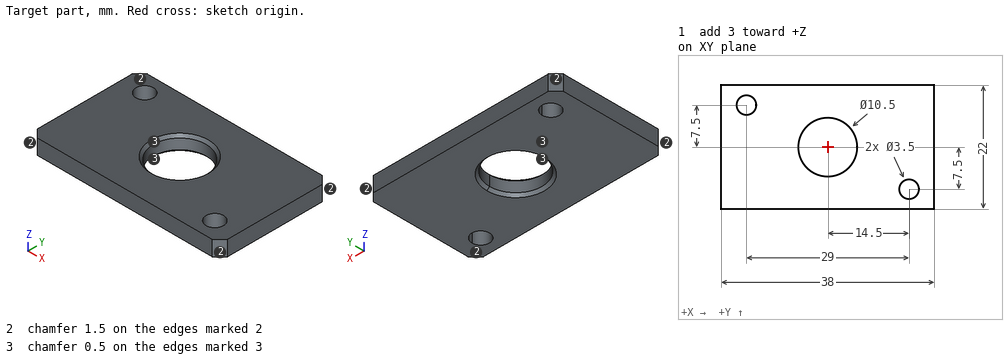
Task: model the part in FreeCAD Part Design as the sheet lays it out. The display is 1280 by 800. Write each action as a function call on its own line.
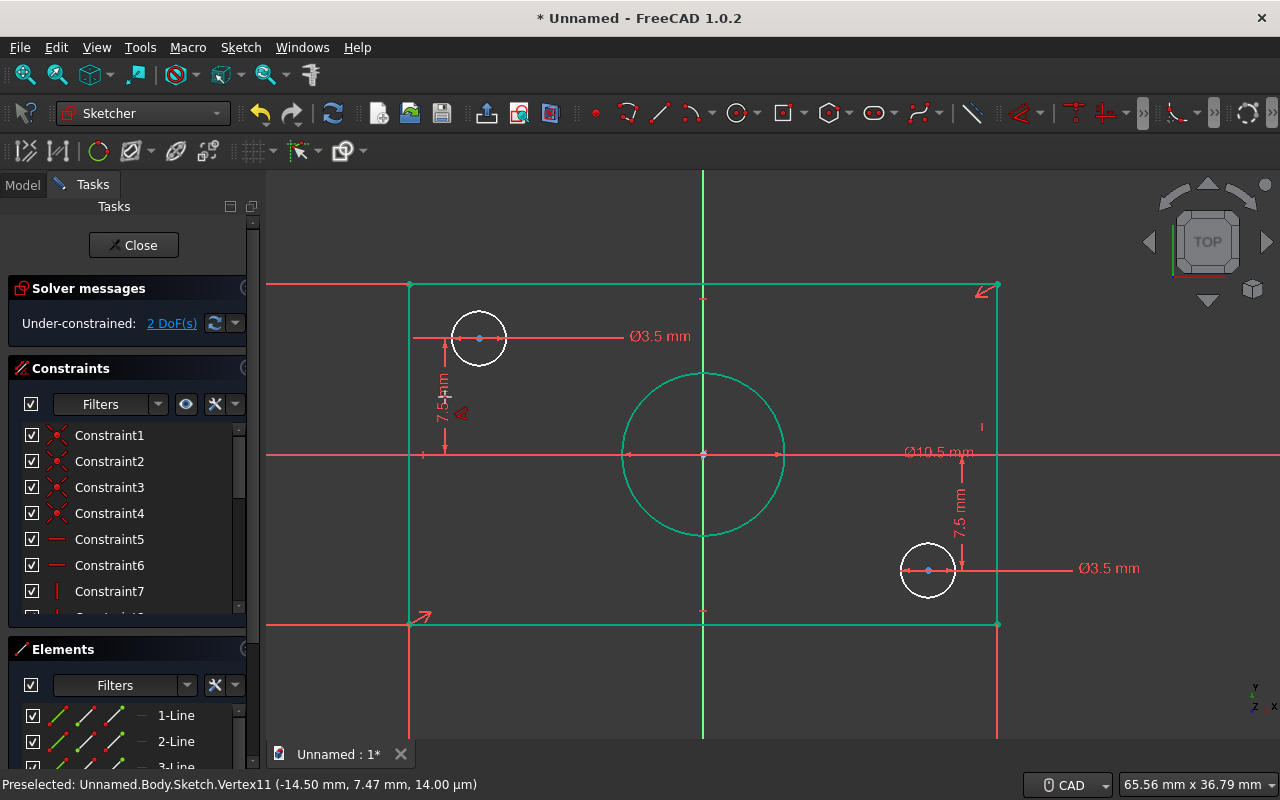
click(928, 571)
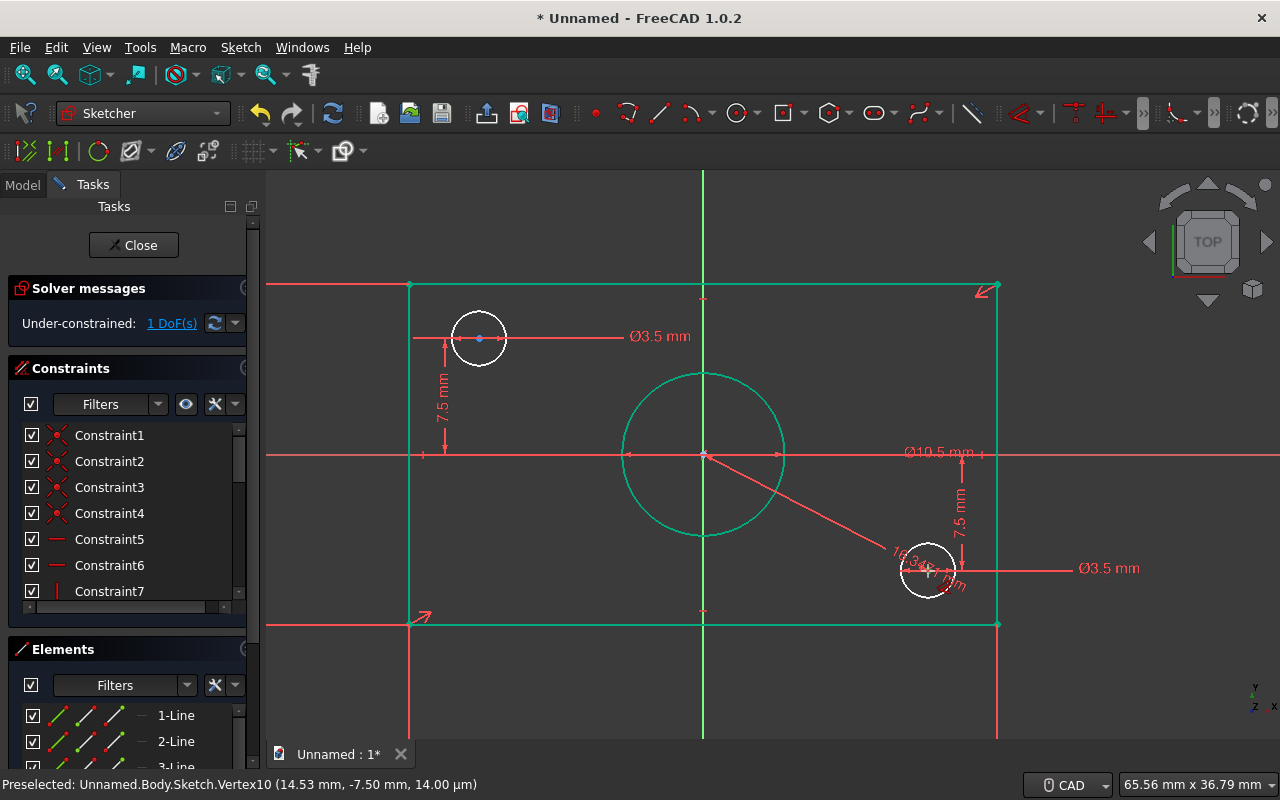
click(479, 338)
click(600, 605)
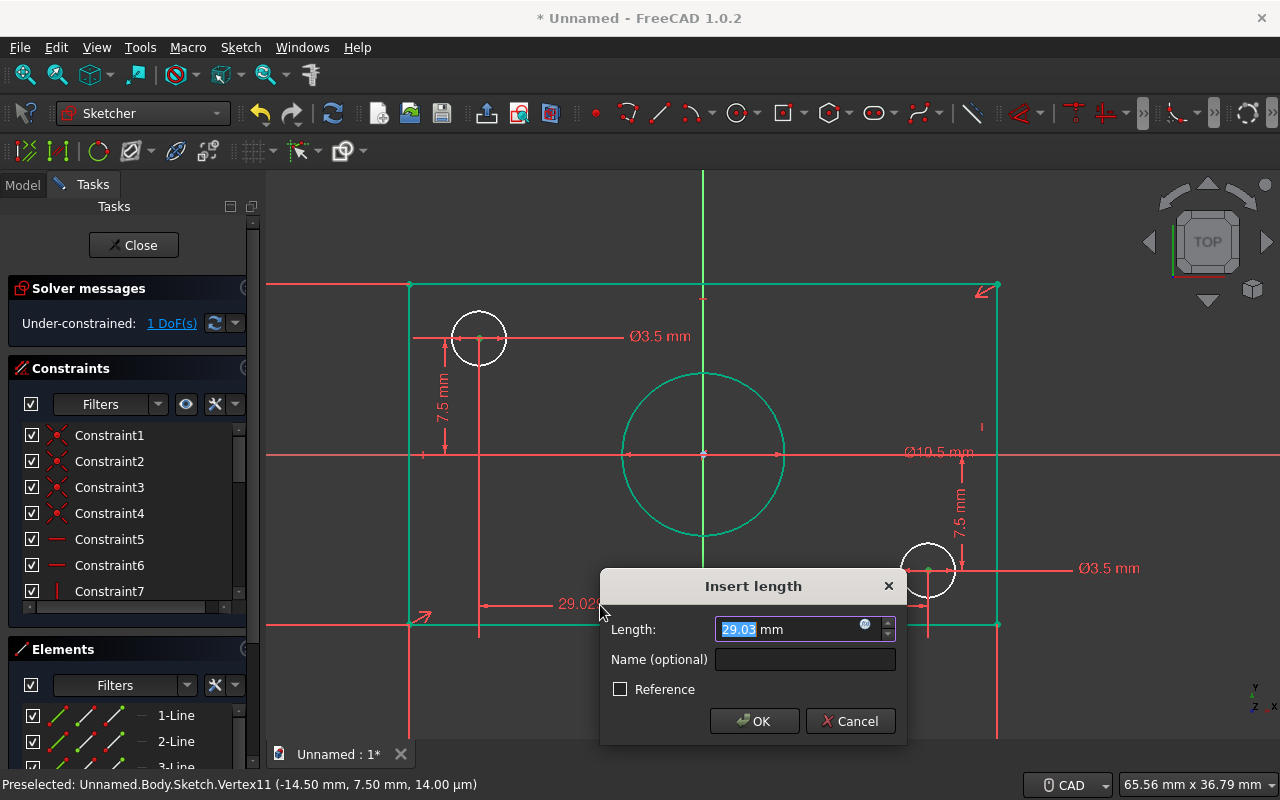
text(29)
key(Return)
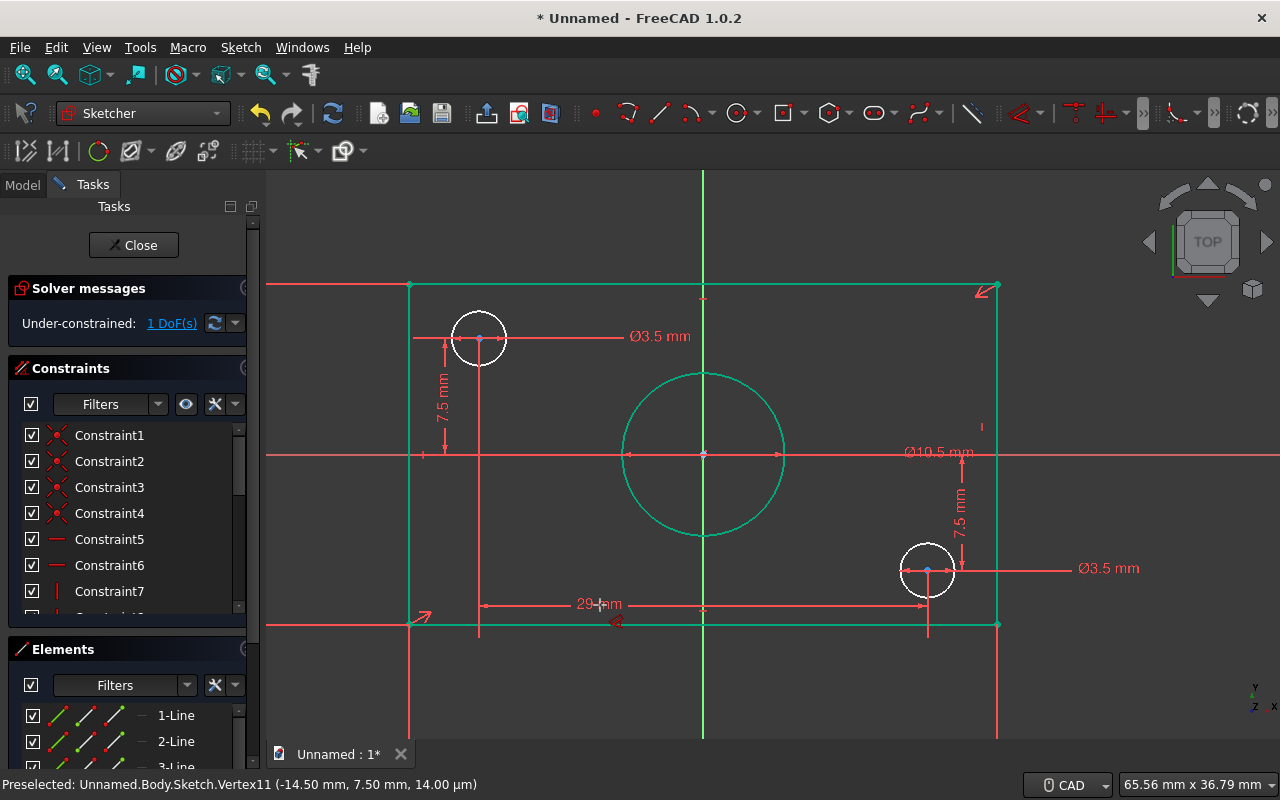
click(928, 571)
click(815, 605)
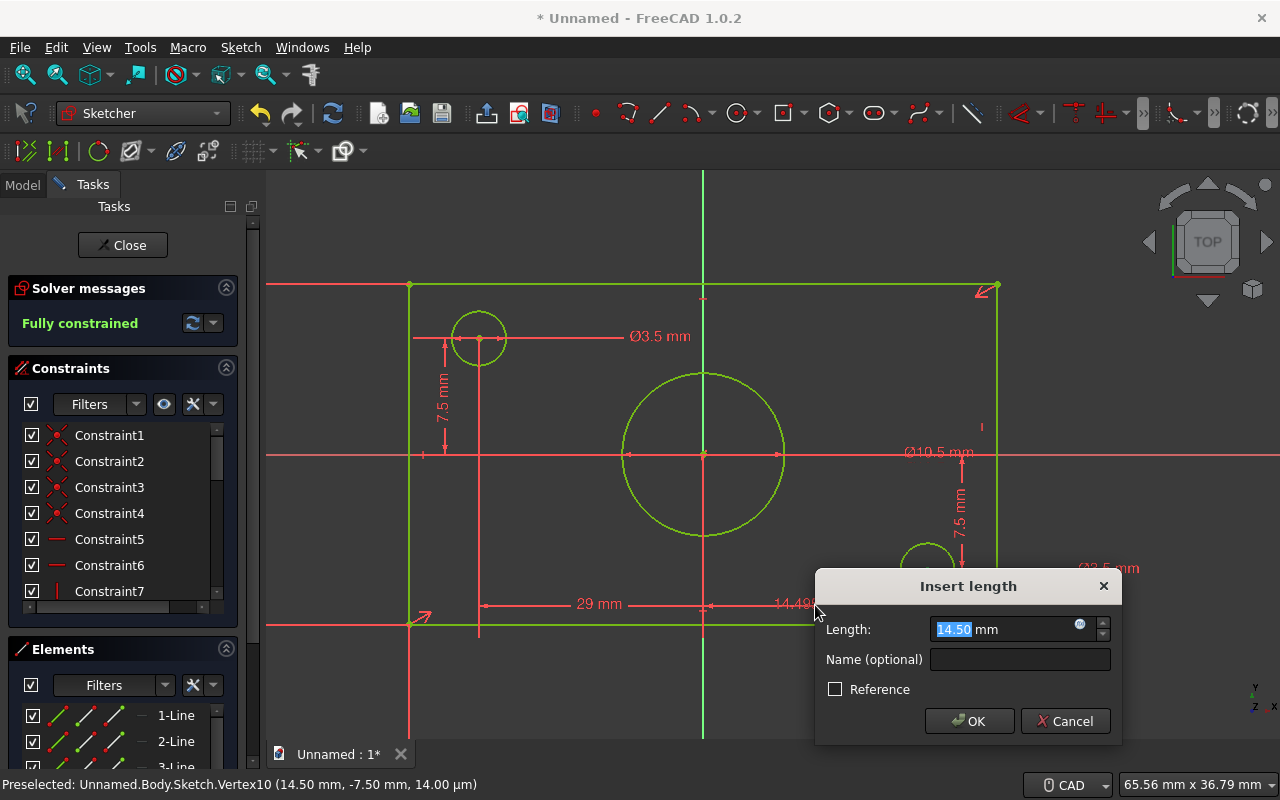
text(14.5)
key(Return)
key(Escape)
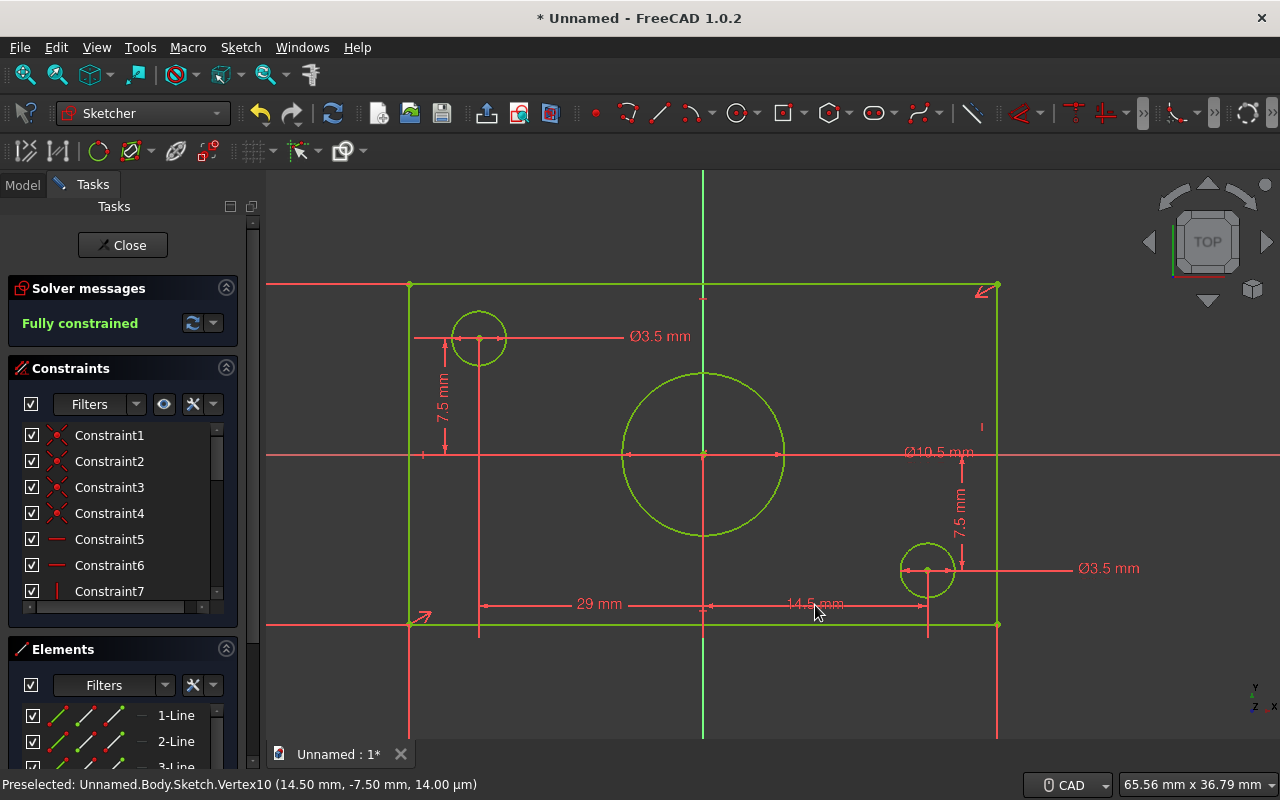
click(123, 245)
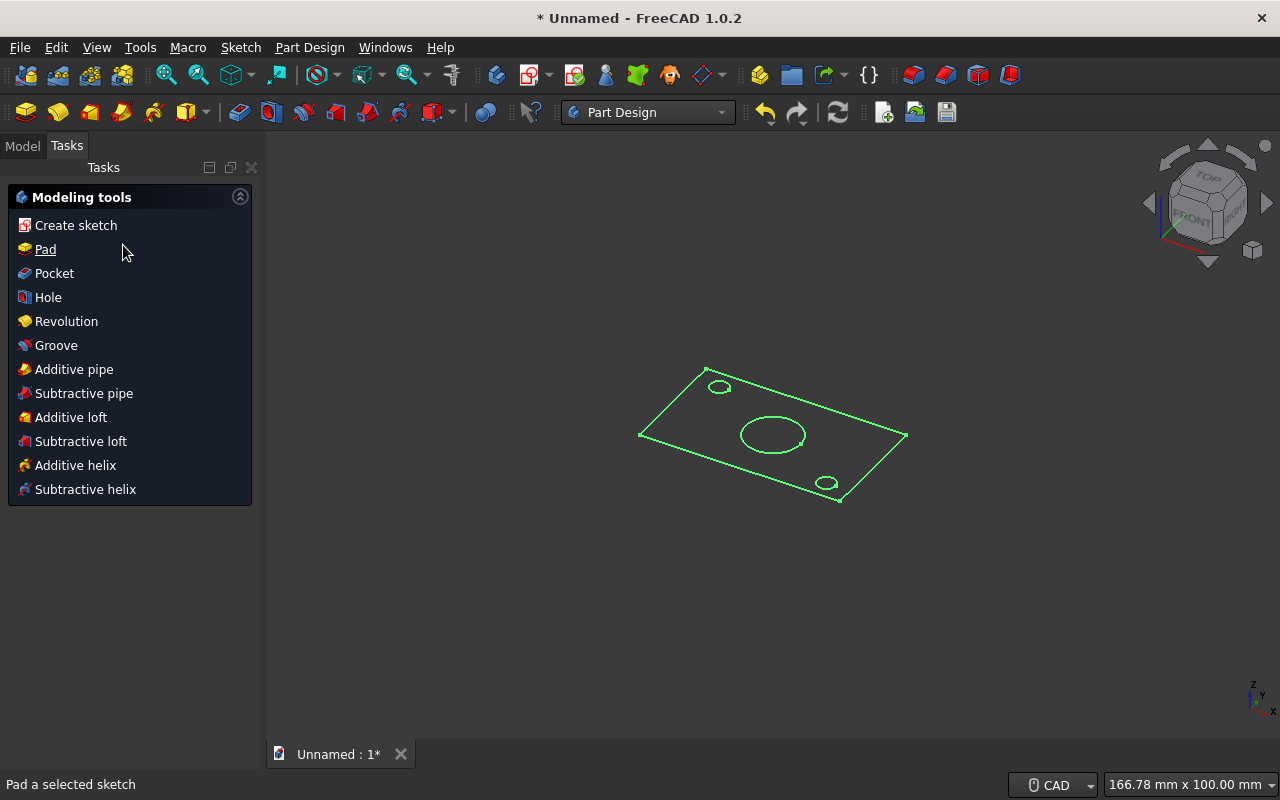
click(26, 112)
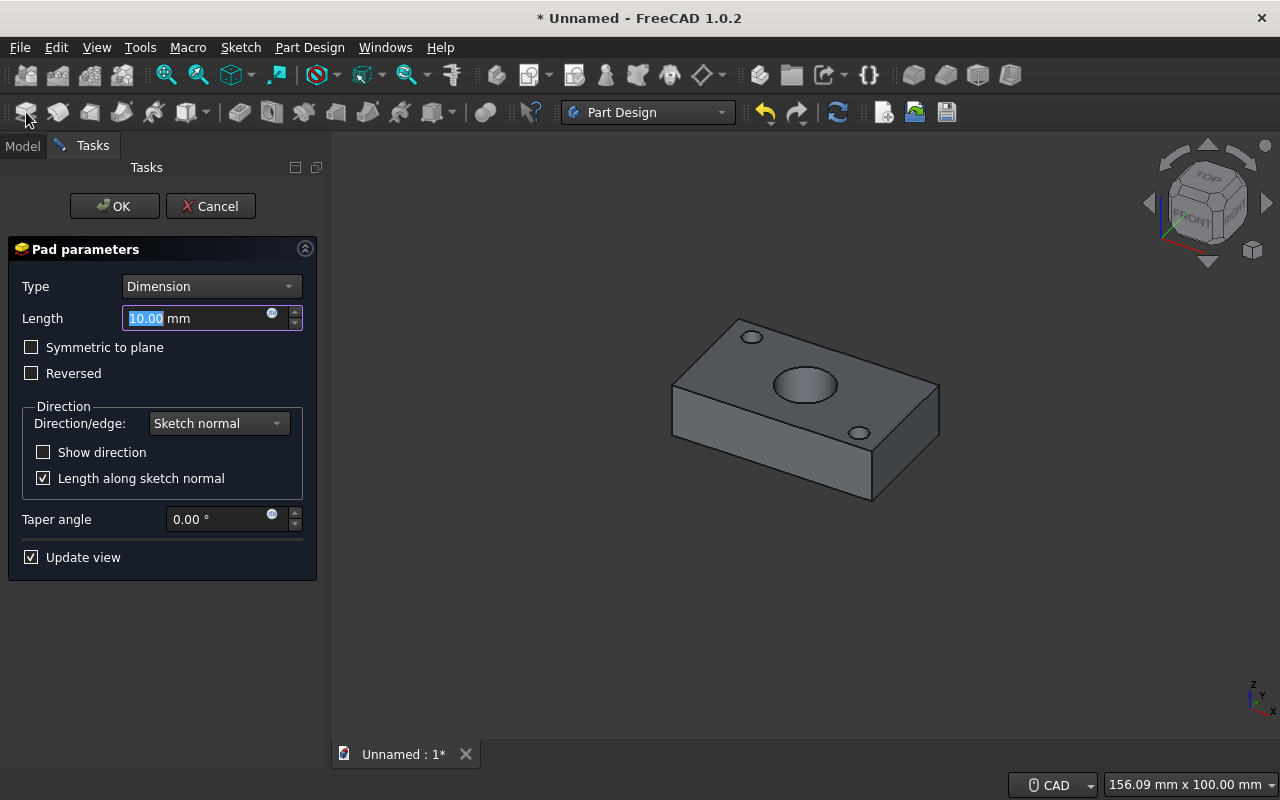
text(3)
key(Tab)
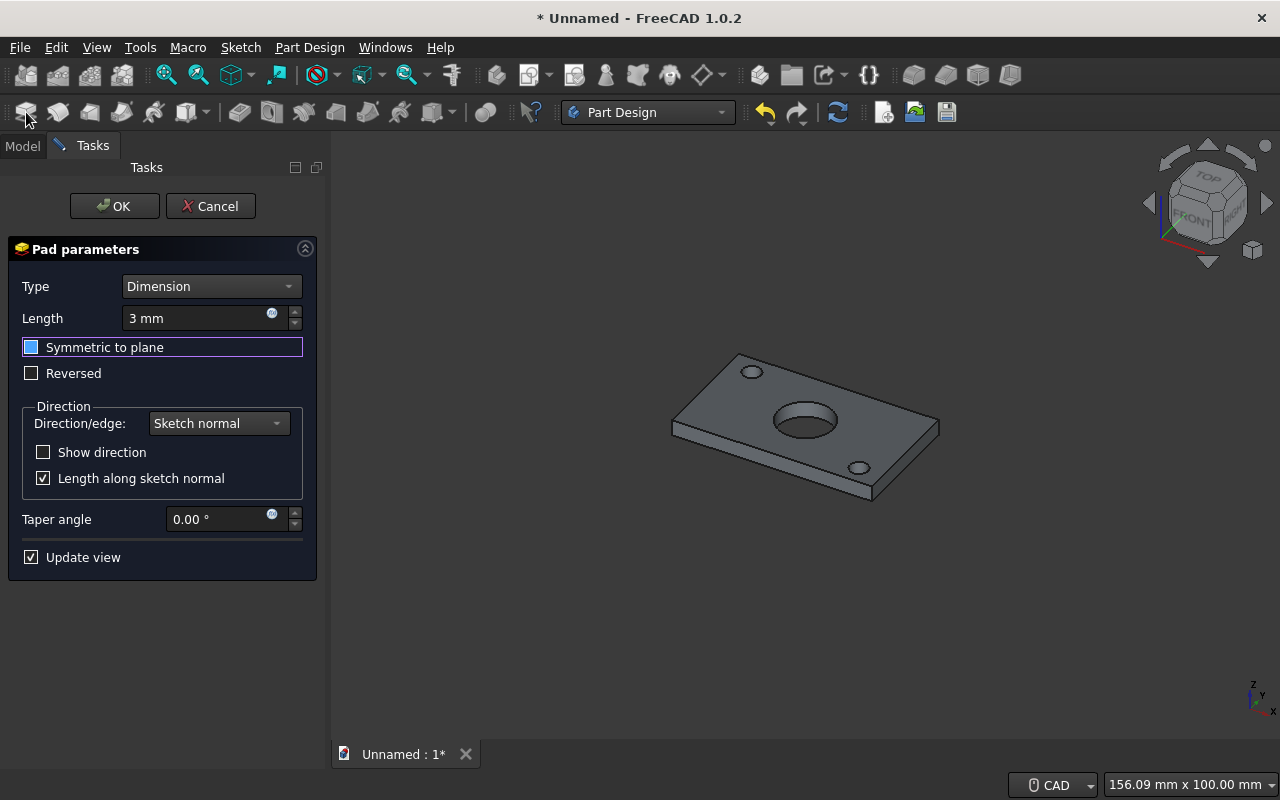
click(115, 206)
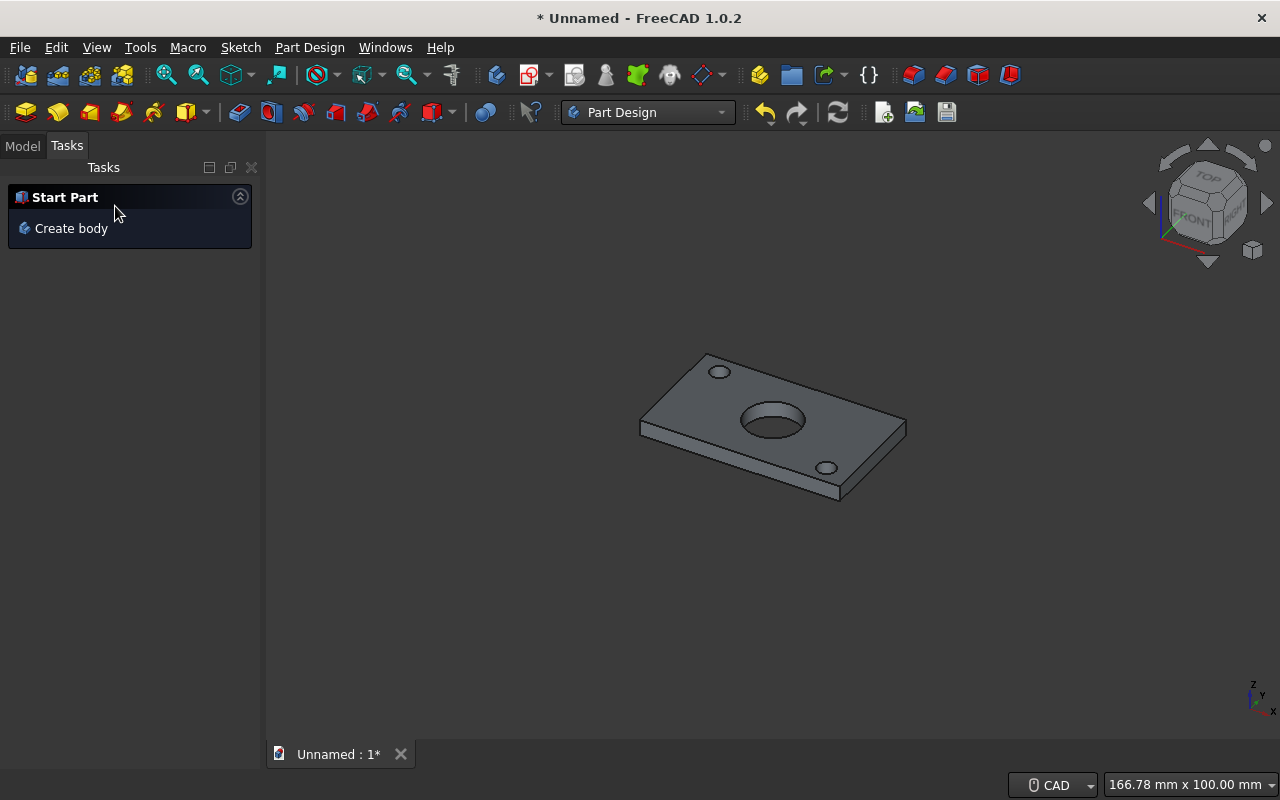
click(168, 76)